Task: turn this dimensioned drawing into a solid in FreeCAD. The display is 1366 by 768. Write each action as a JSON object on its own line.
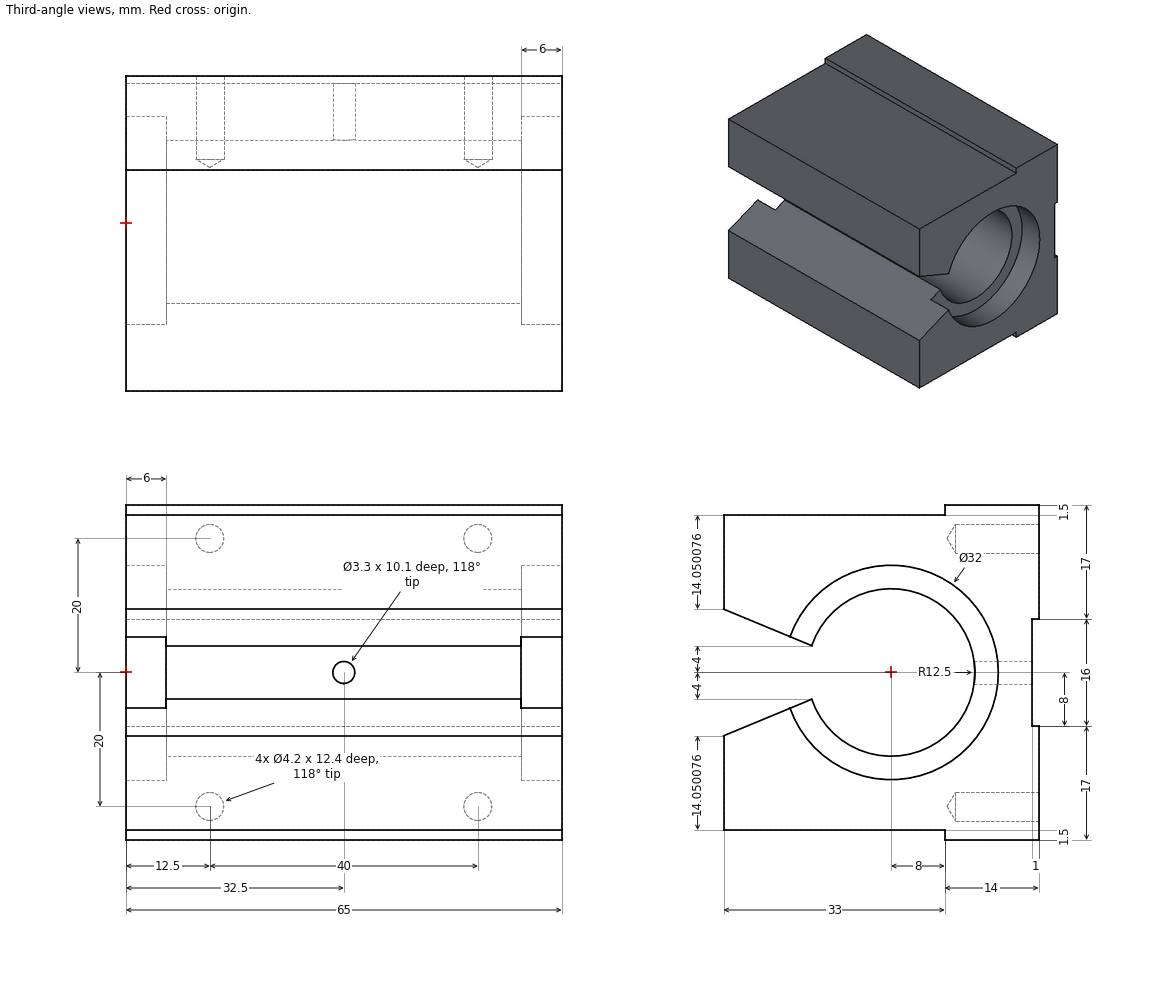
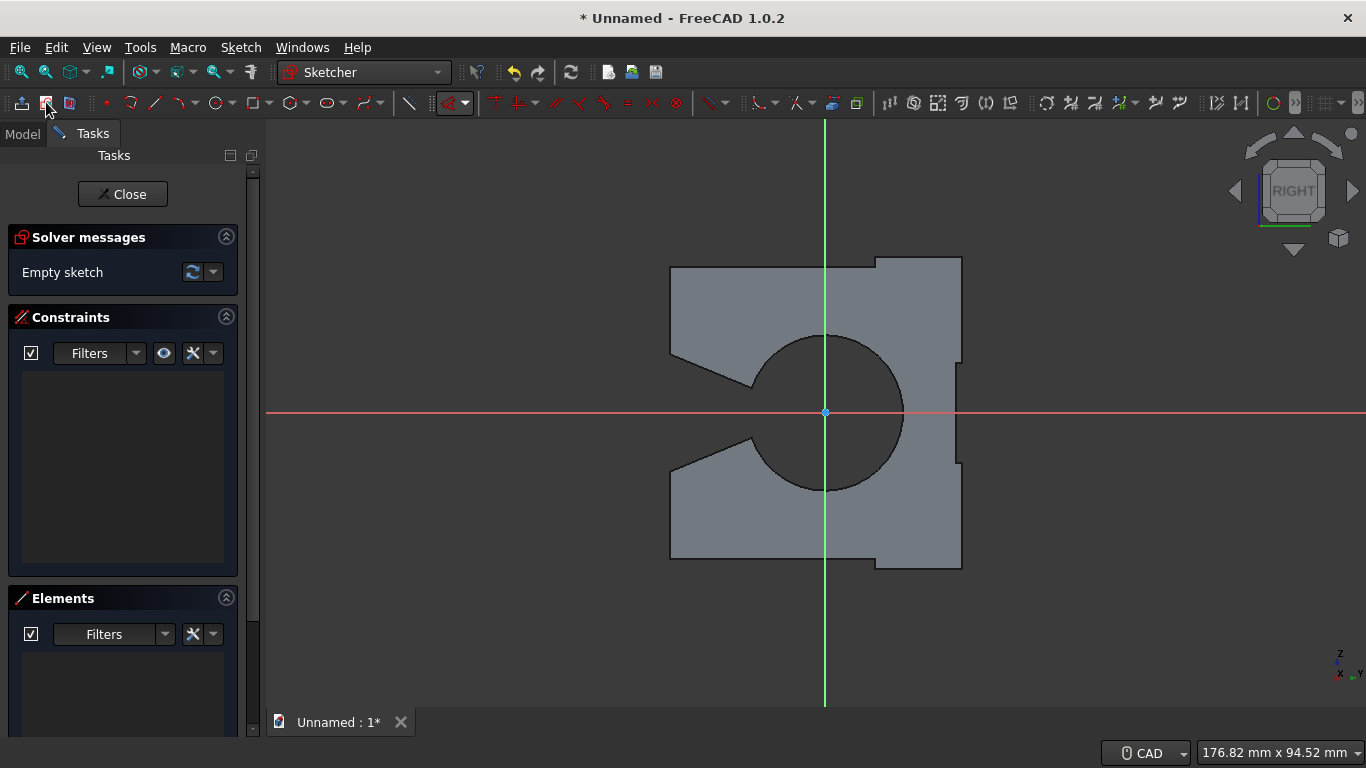
{"action": "scroll", "coordinate": [920, 413], "scroll_direction": "up", "scroll_amount": 3}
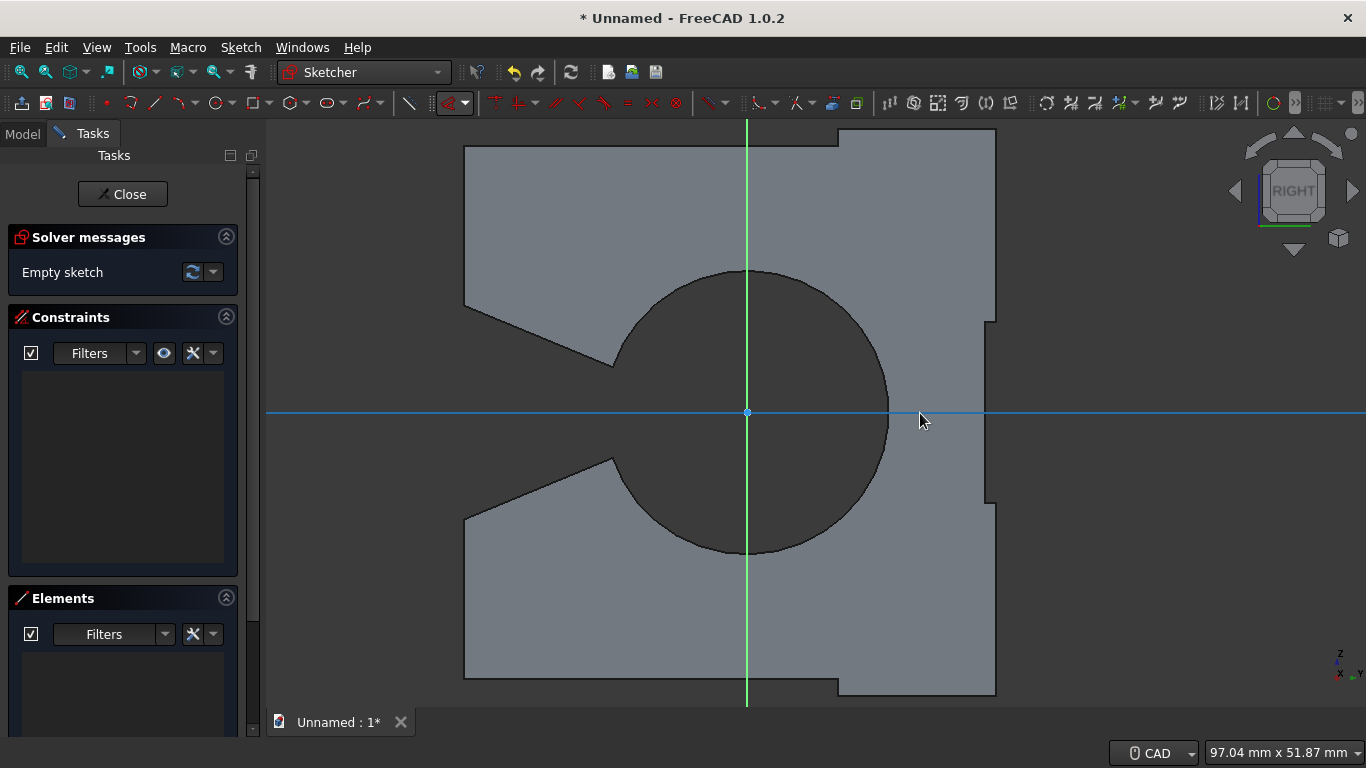
{"action": "key", "text": "g c"}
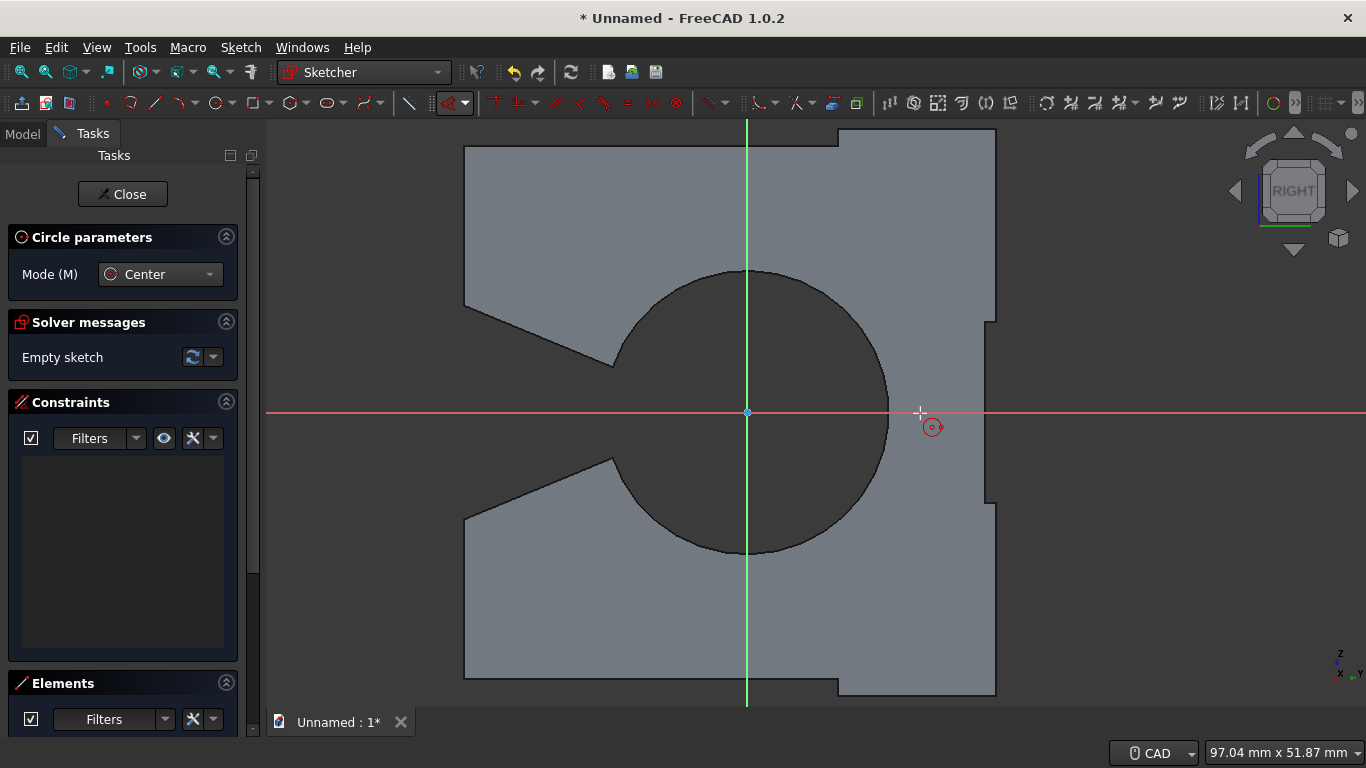
{"action": "left_click", "coordinate": [747, 413]}
{"action": "left_click", "coordinate": [875, 284]}
{"action": "key", "text": "Escape"}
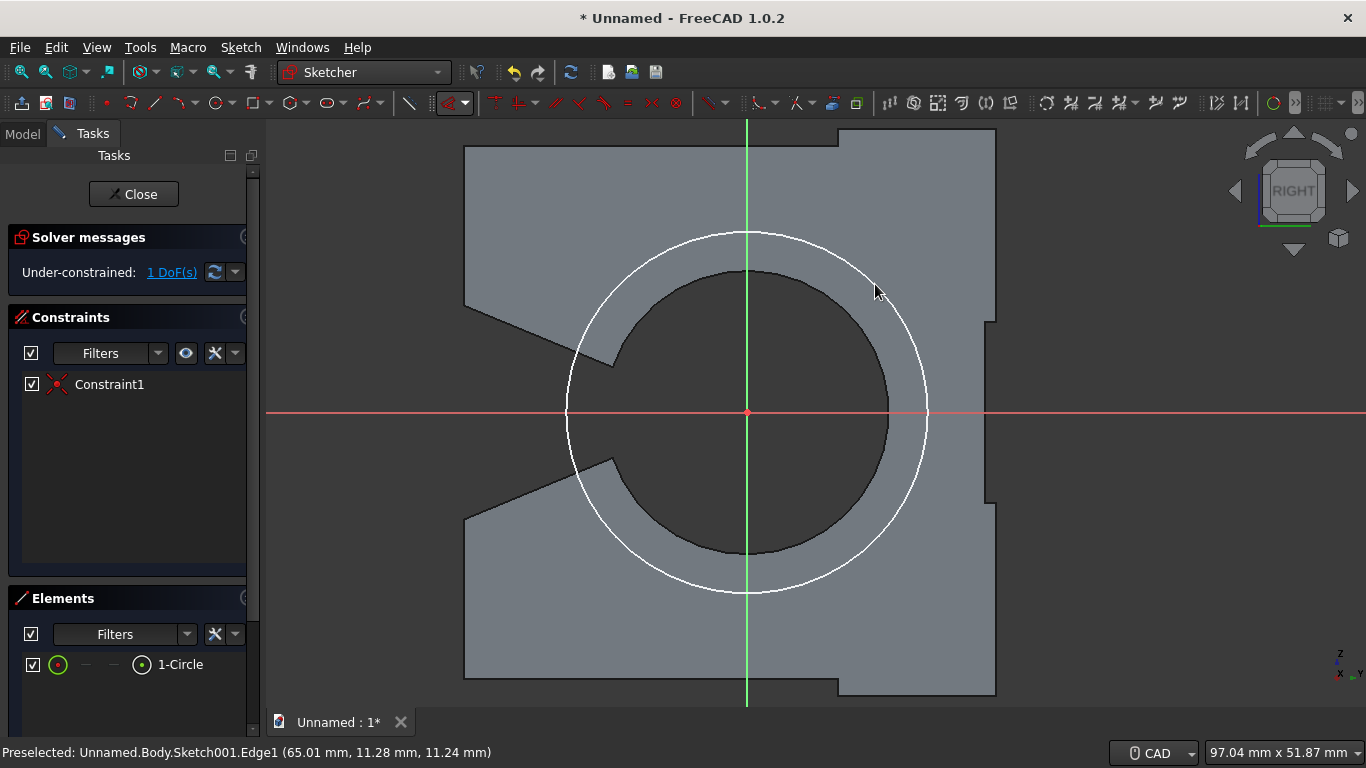
{"action": "left_click", "coordinate": [874, 284]}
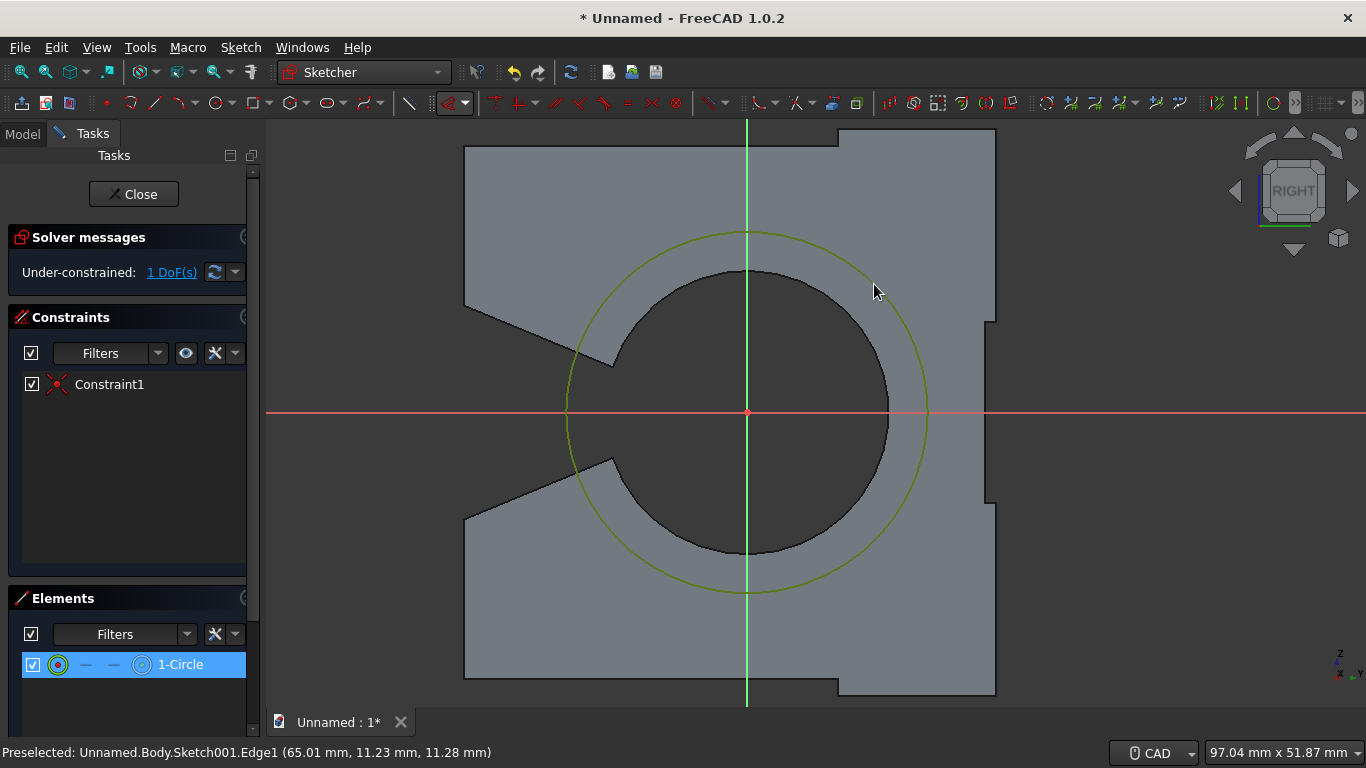
{"action": "key", "text": "k o"}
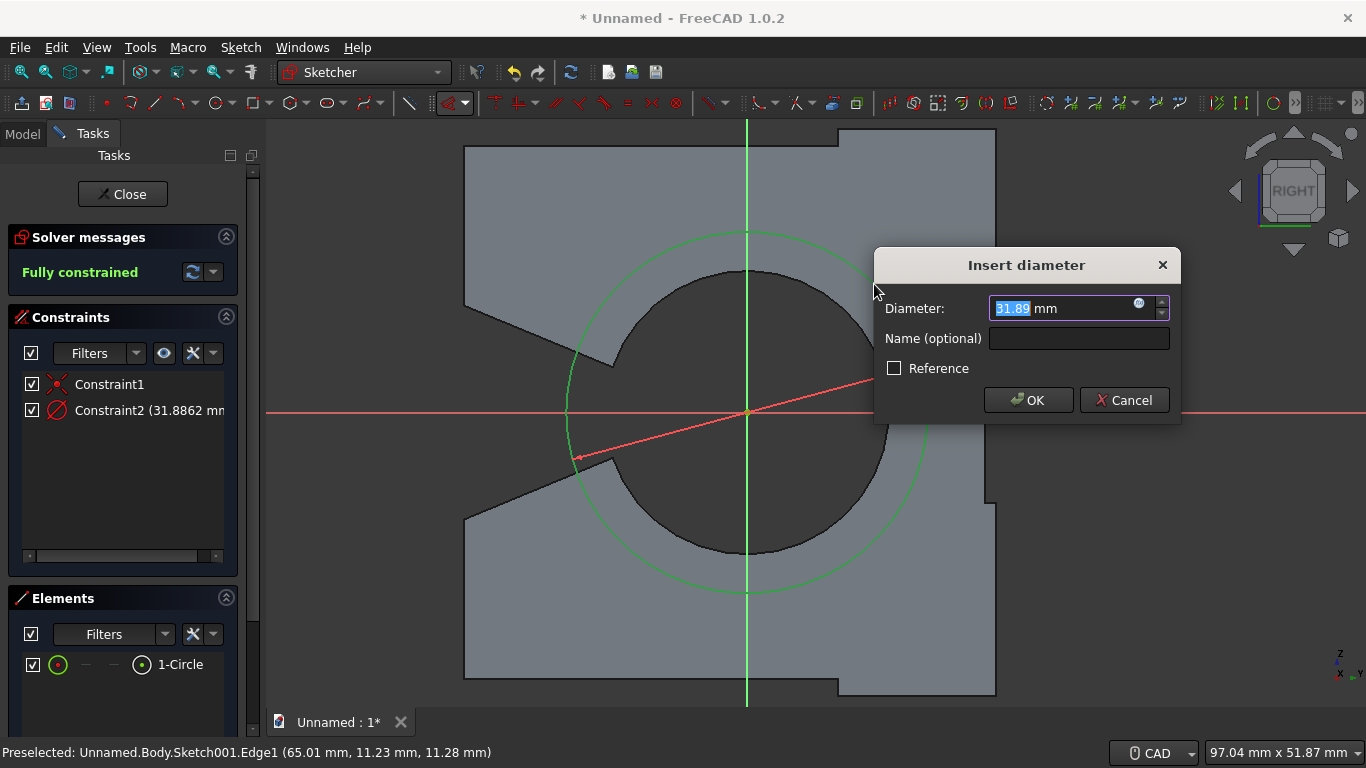
{"action": "type", "text": "32"}
{"action": "key", "text": "Return"}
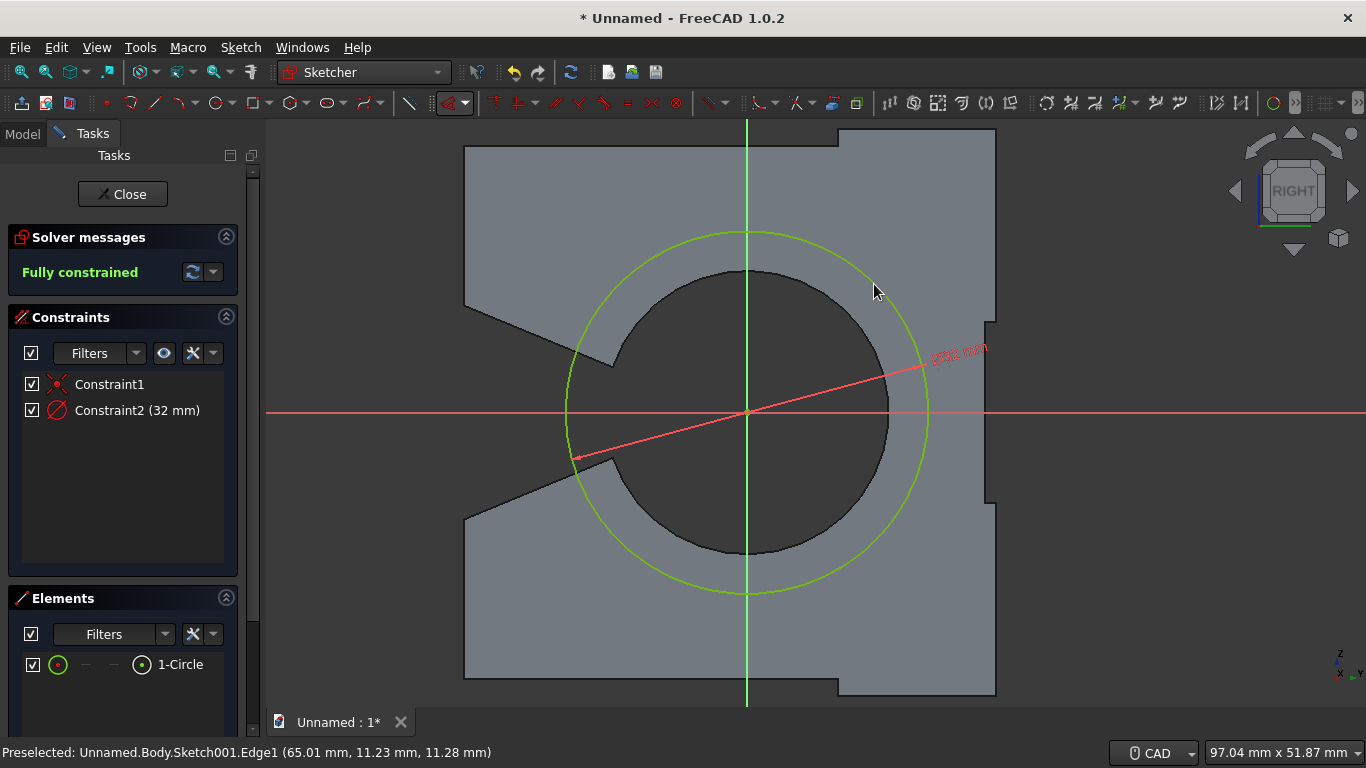
{"action": "left_click", "coordinate": [123, 194]}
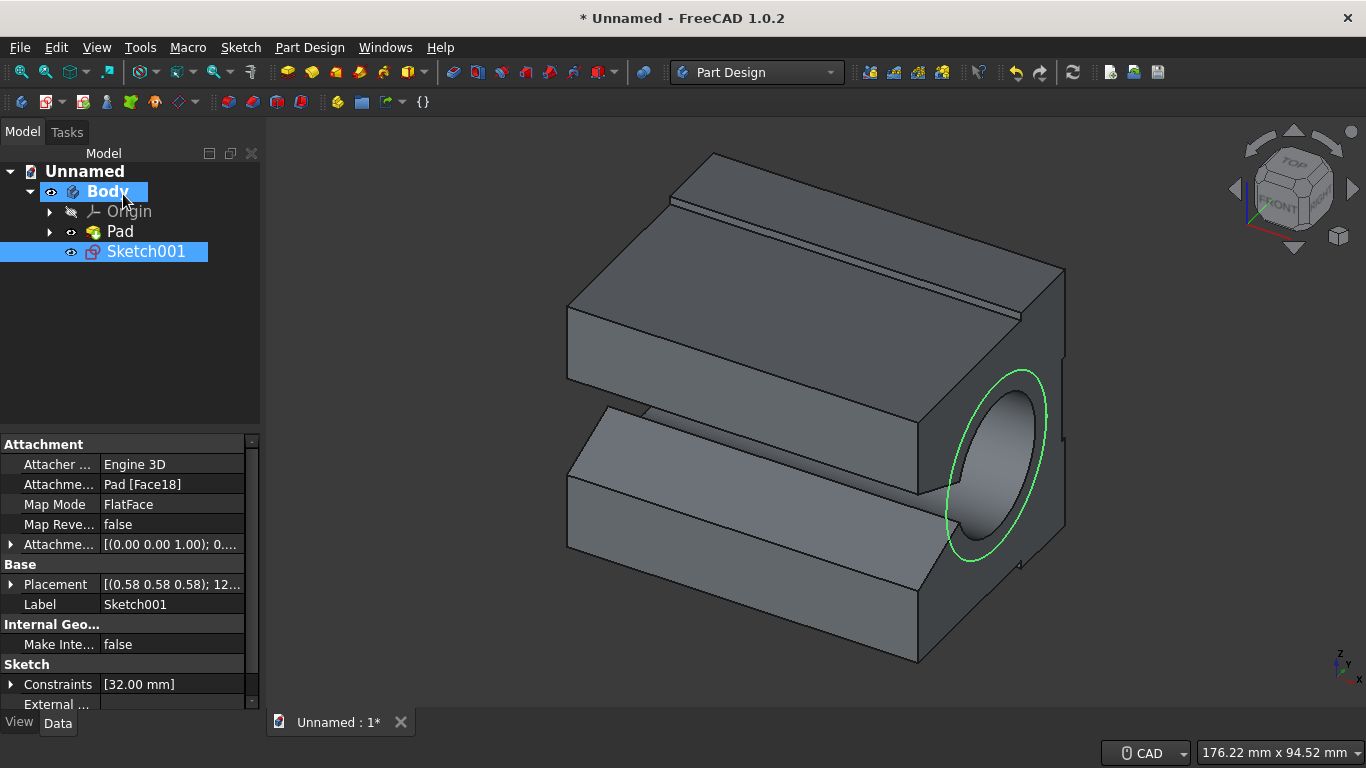
{"action": "left_click", "coordinate": [454, 72]}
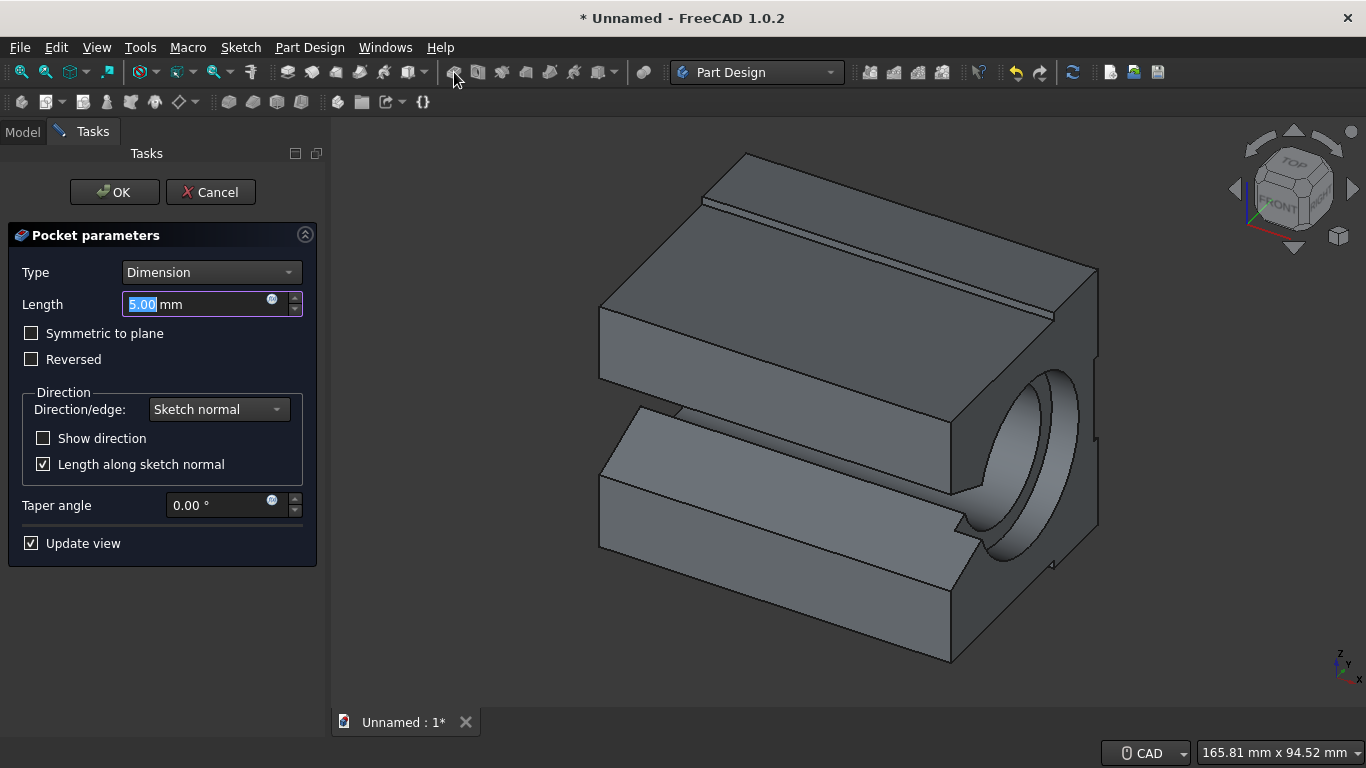
{"action": "type", "text": "6"}
{"action": "key", "text": "Tab"}